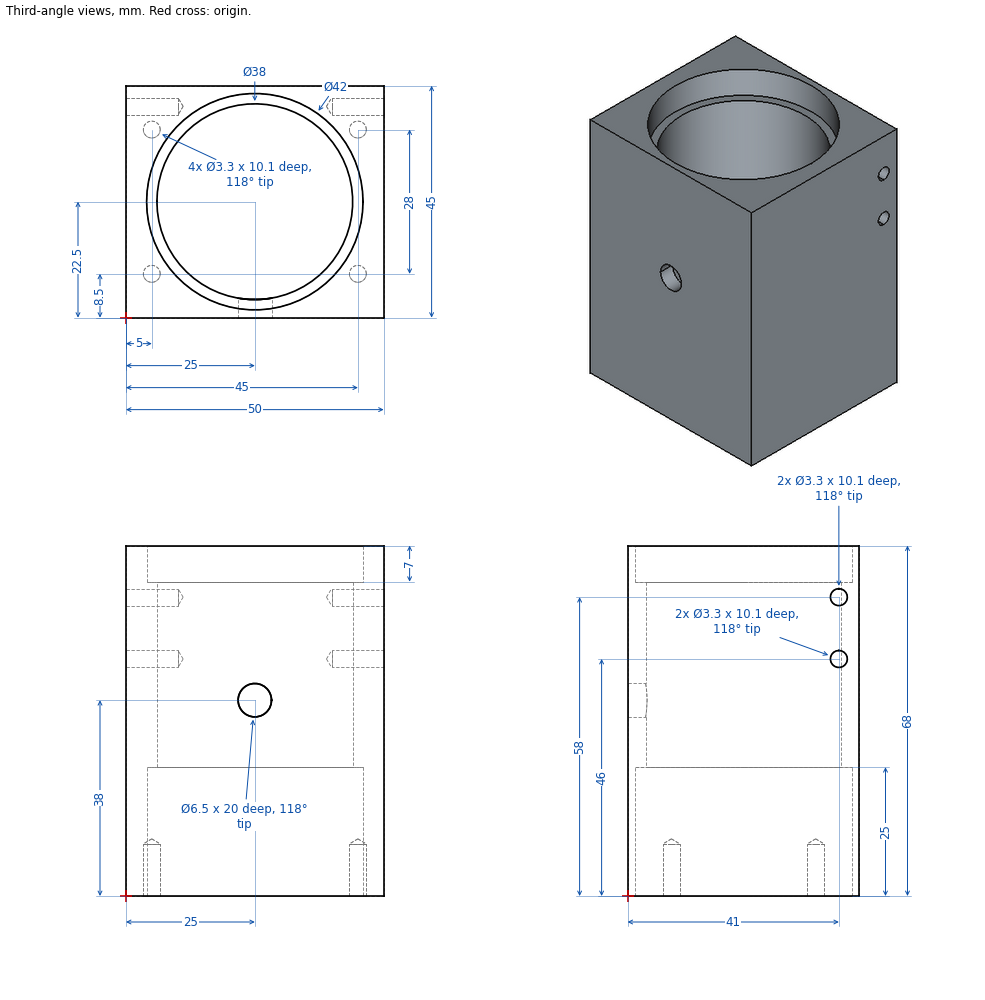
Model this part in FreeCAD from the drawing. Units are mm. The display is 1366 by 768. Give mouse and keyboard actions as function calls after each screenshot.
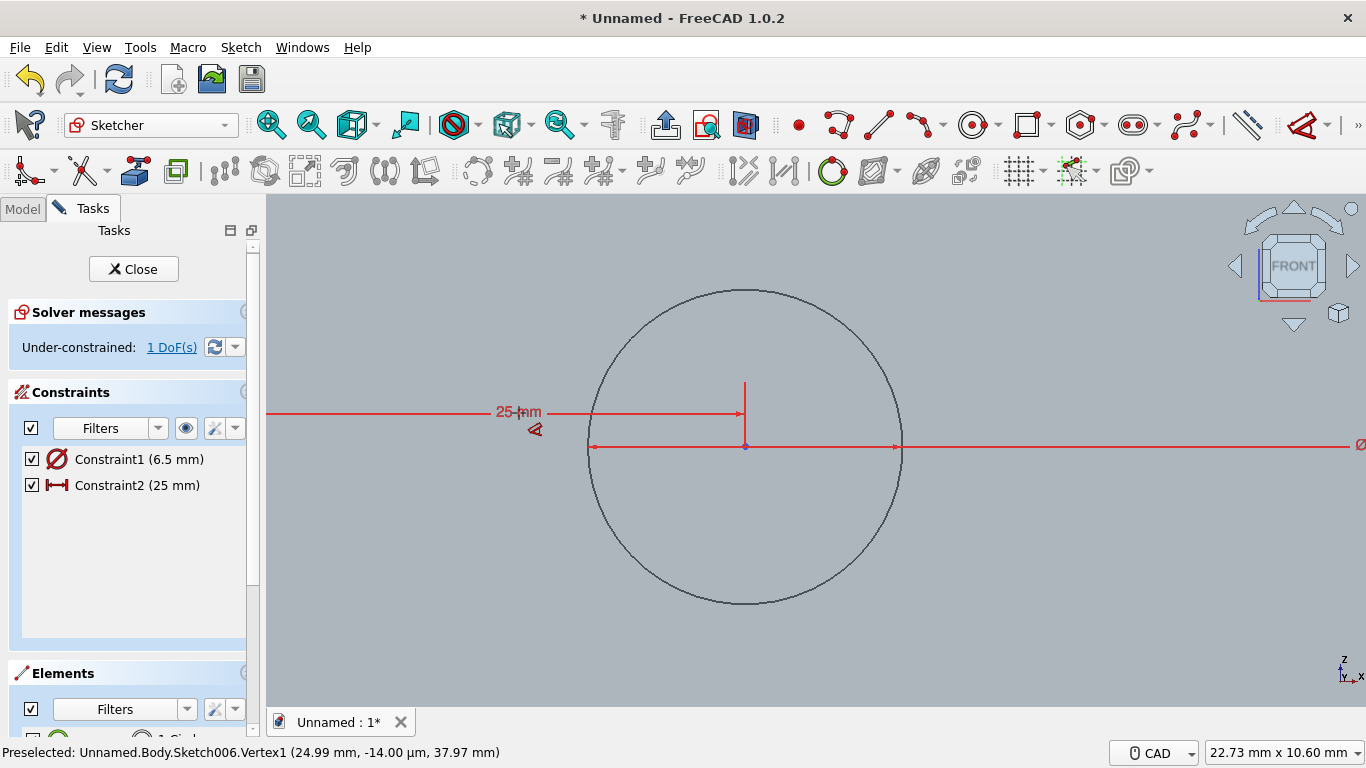
click(745, 447)
click(779, 563)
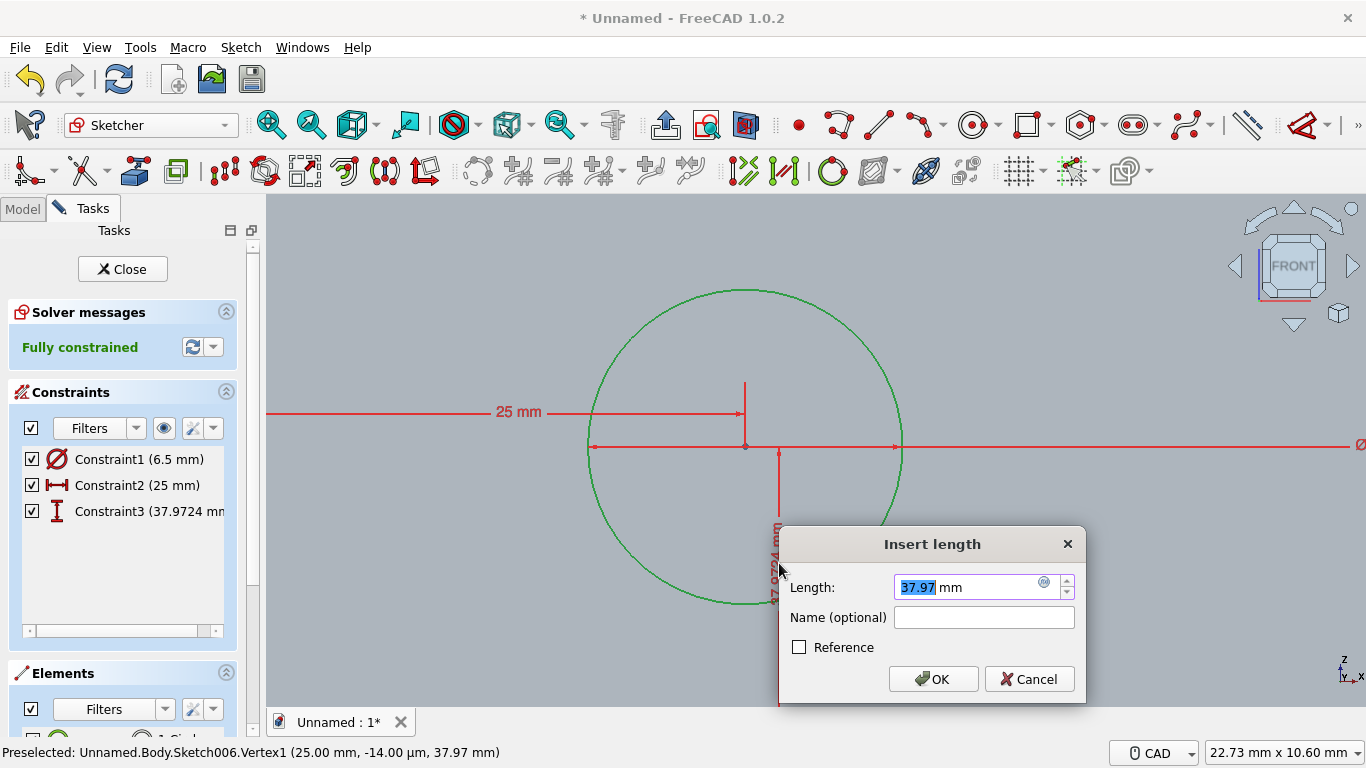
text(38)
key(Return)
key(Escape)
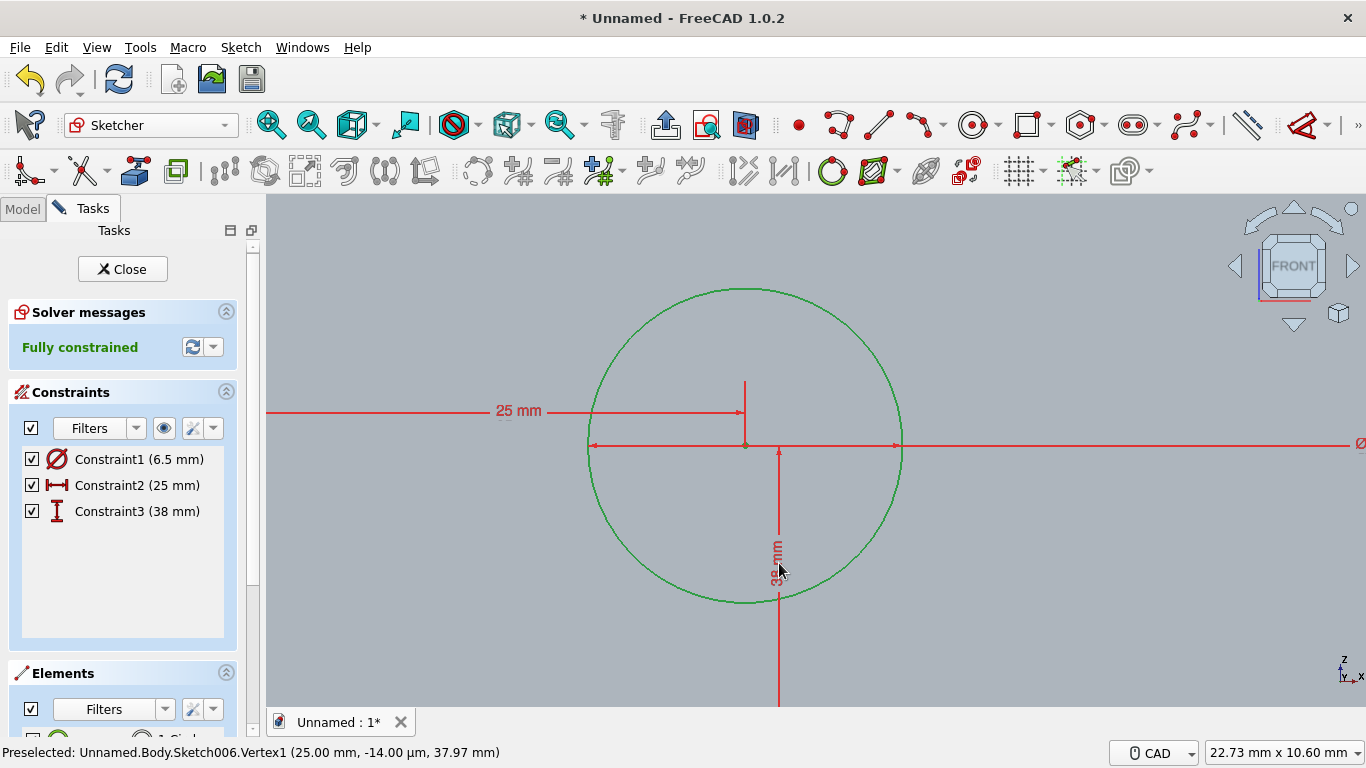
click(123, 269)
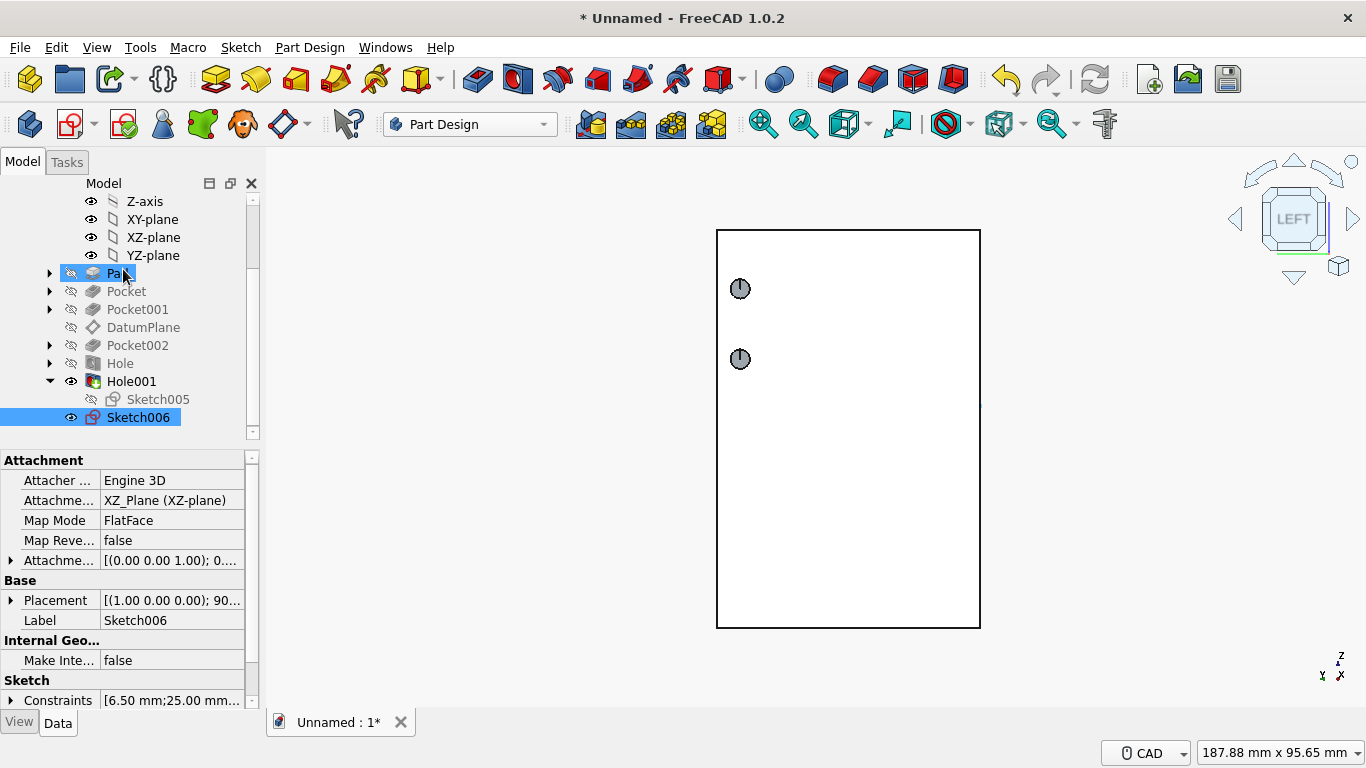
click(518, 80)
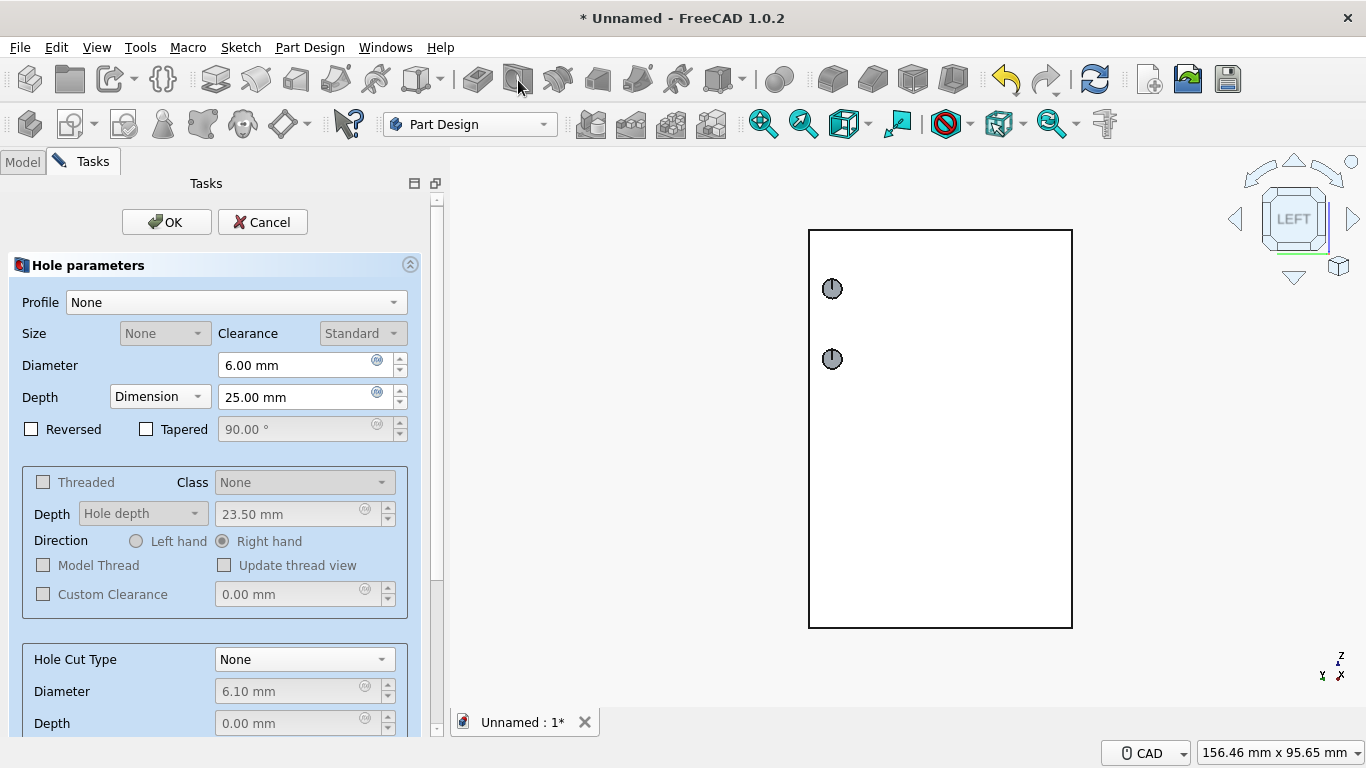
triple_click(305, 365)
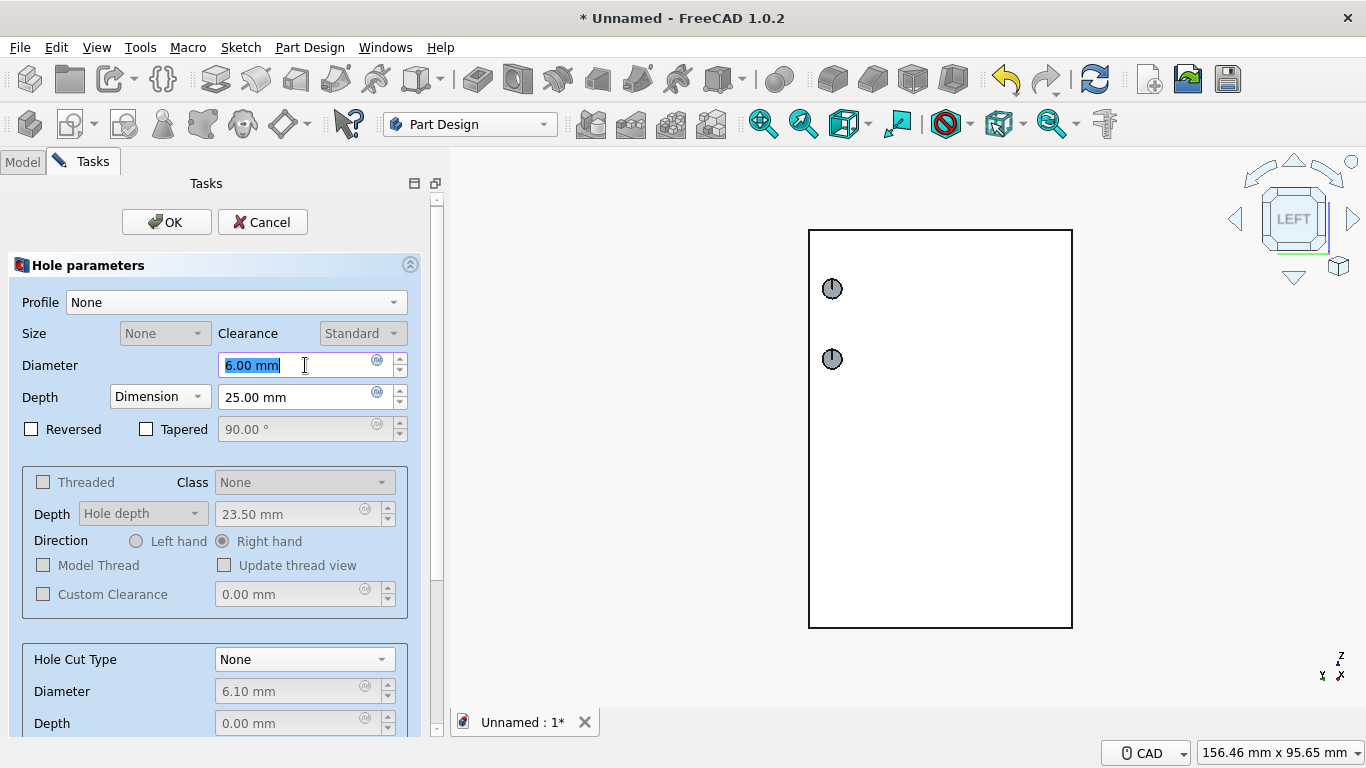
text(6.5)
key(Tab)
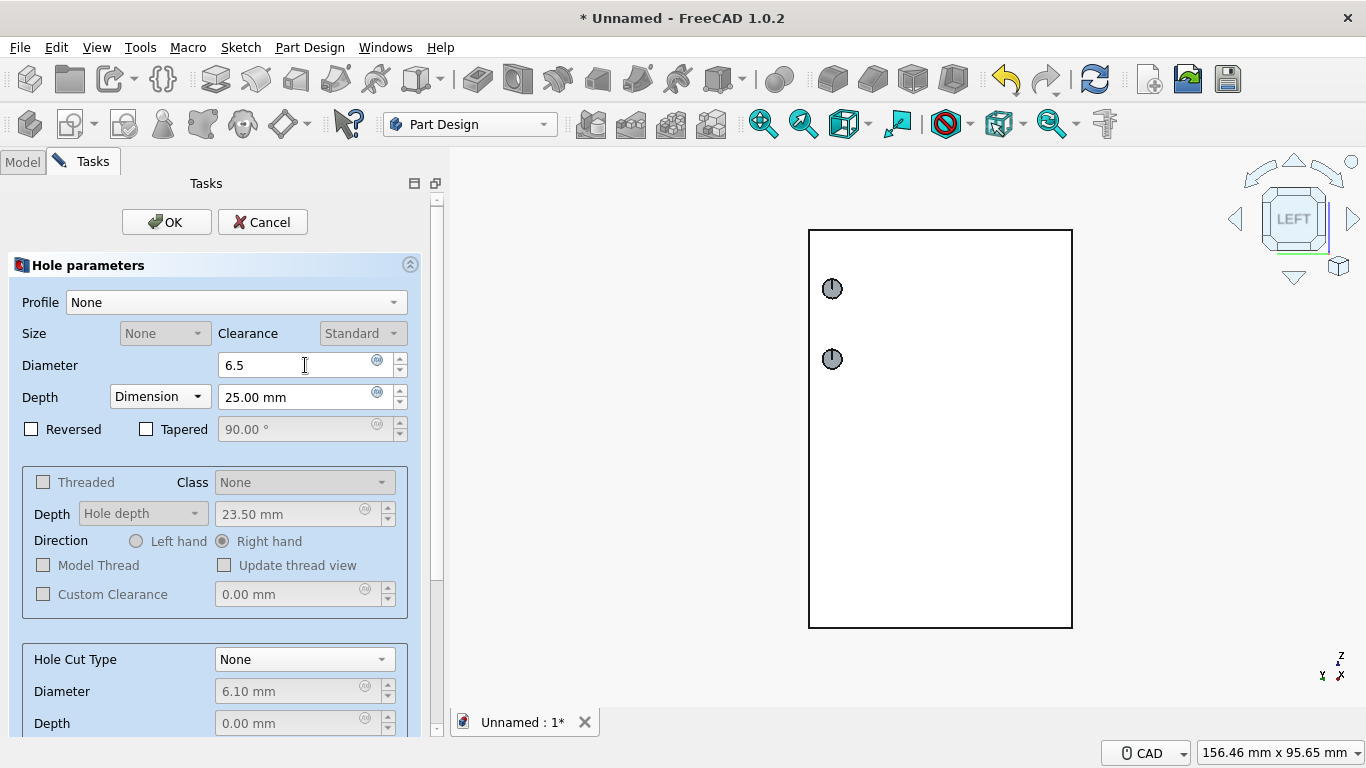
triple_click(305, 397)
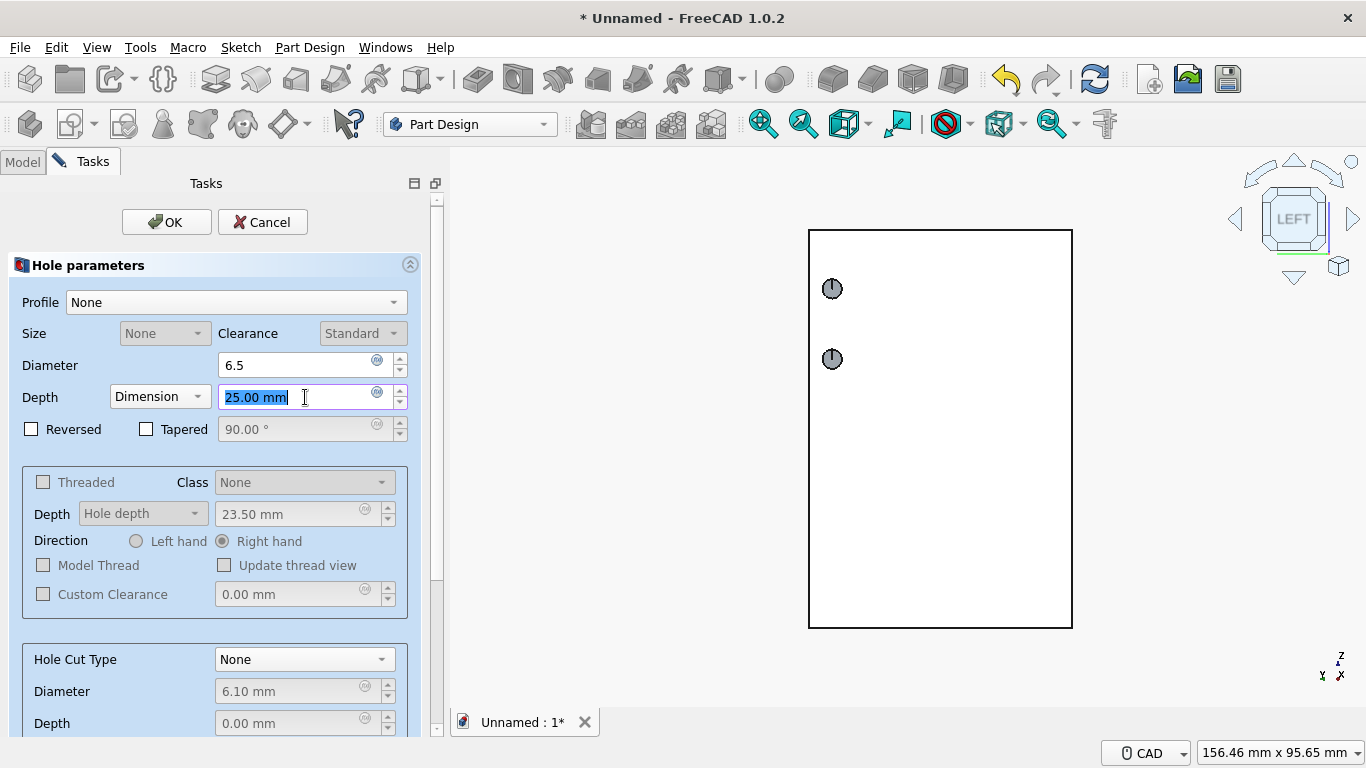
text(20)
key(Tab)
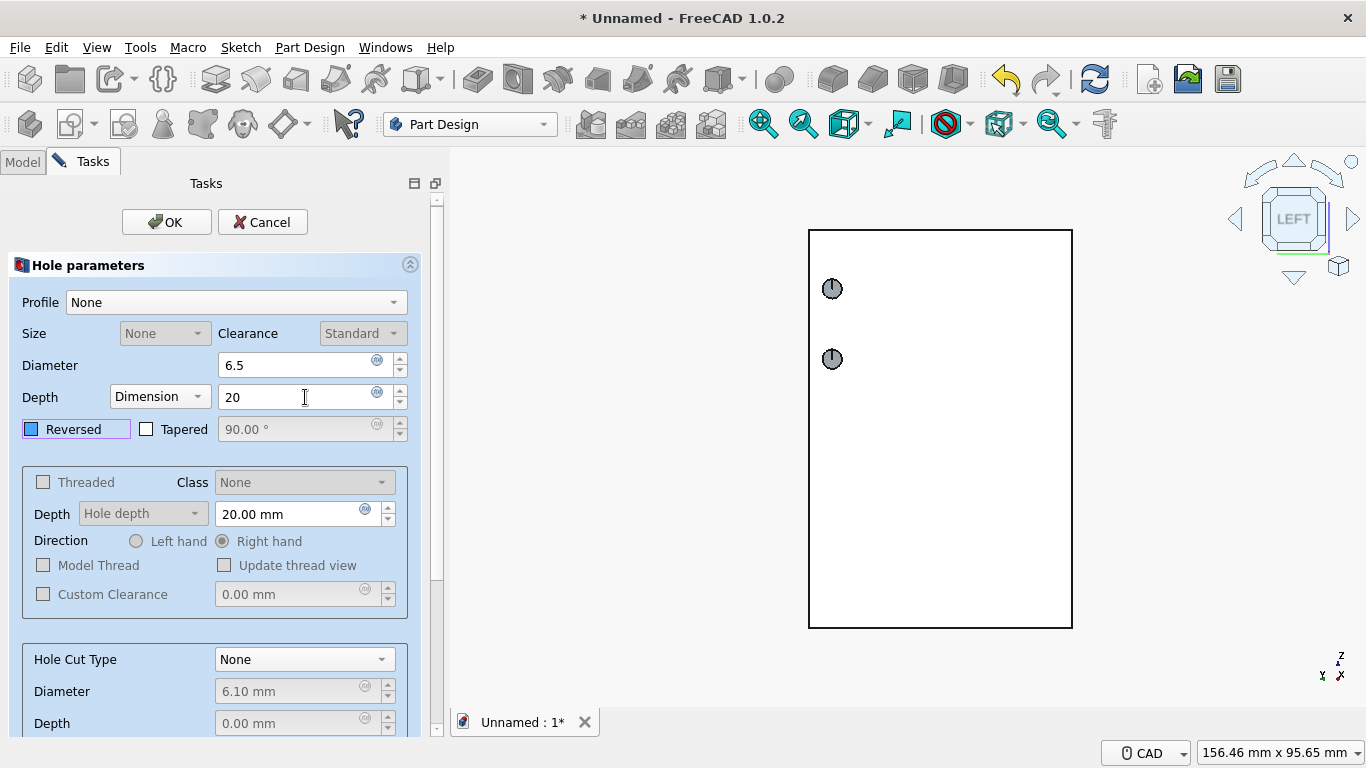
click(167, 222)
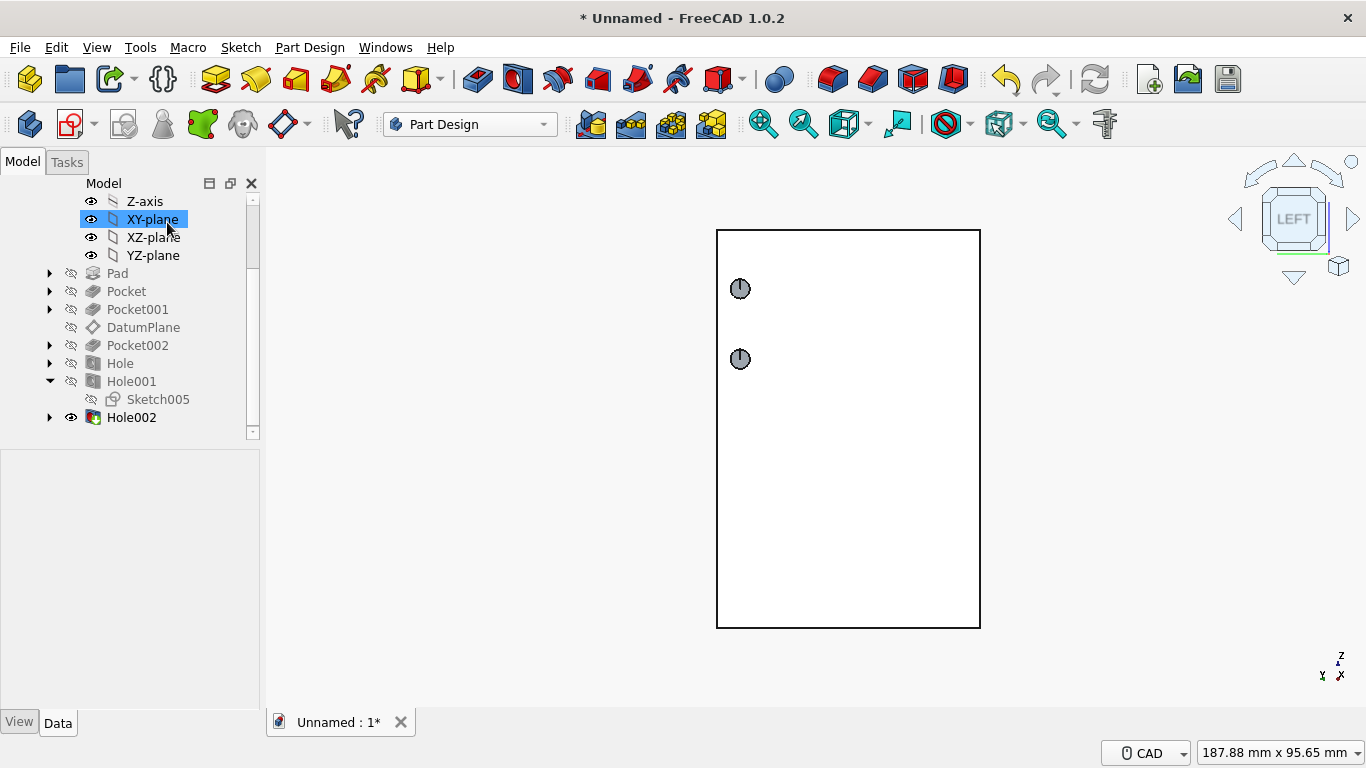
key(5)